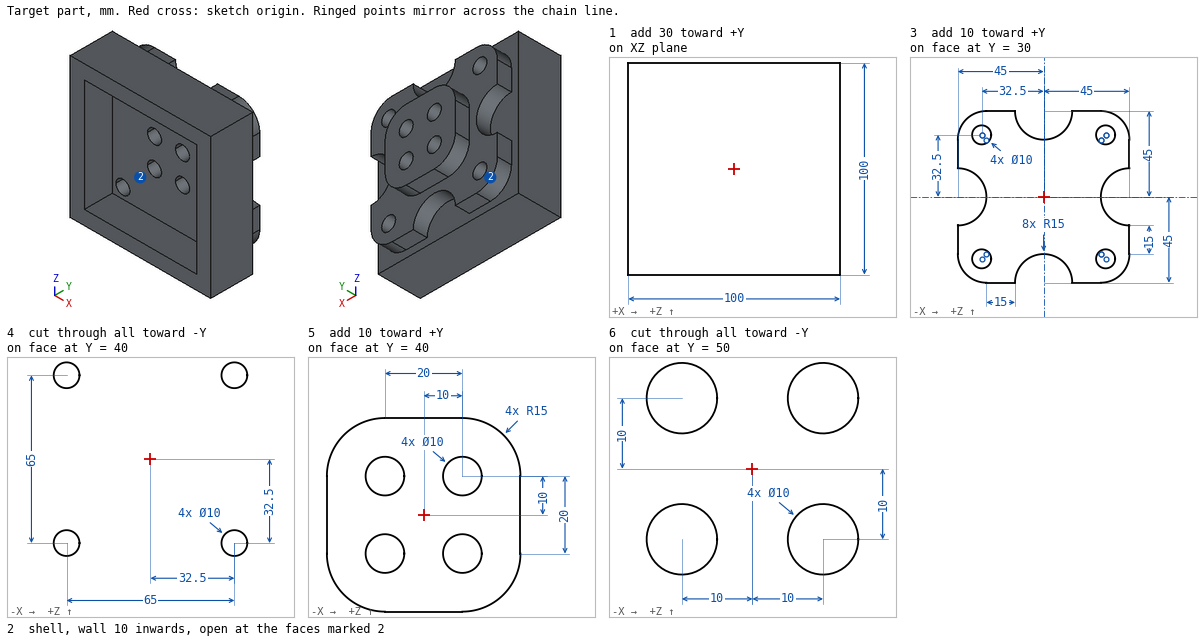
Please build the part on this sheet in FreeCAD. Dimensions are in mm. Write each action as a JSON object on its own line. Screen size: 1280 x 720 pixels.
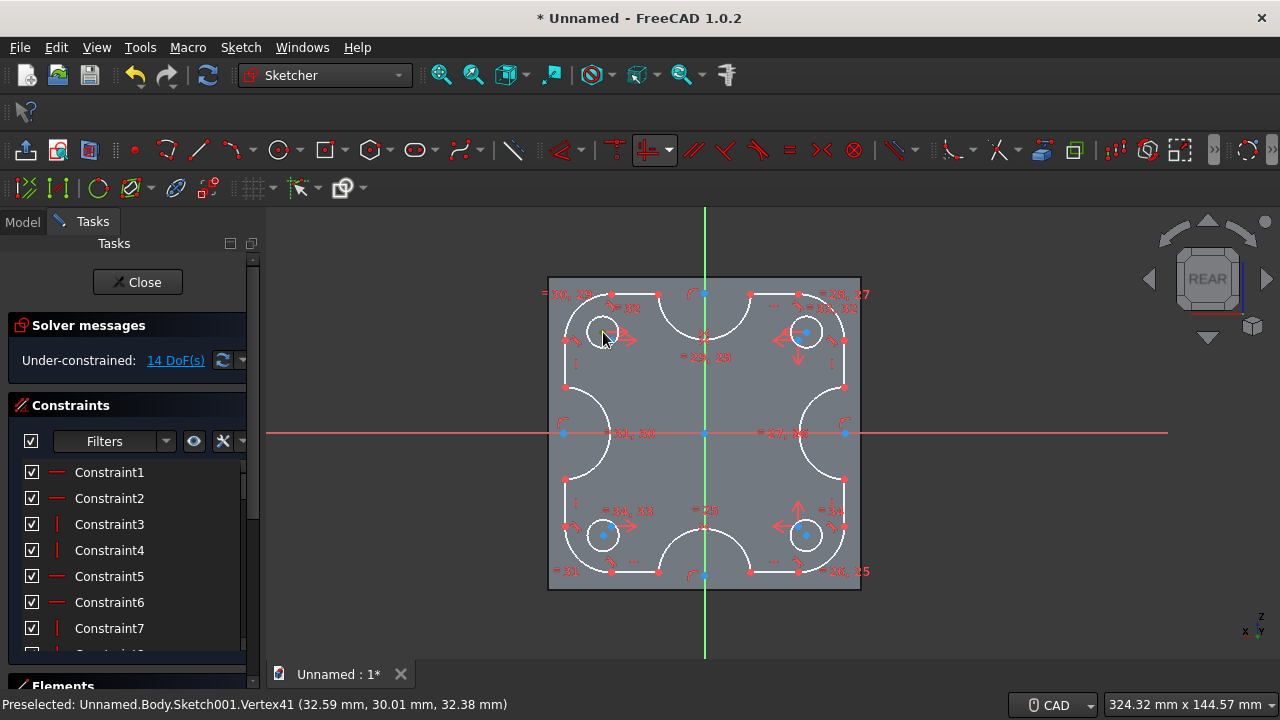
{"action": "left_click", "coordinate": [603, 536]}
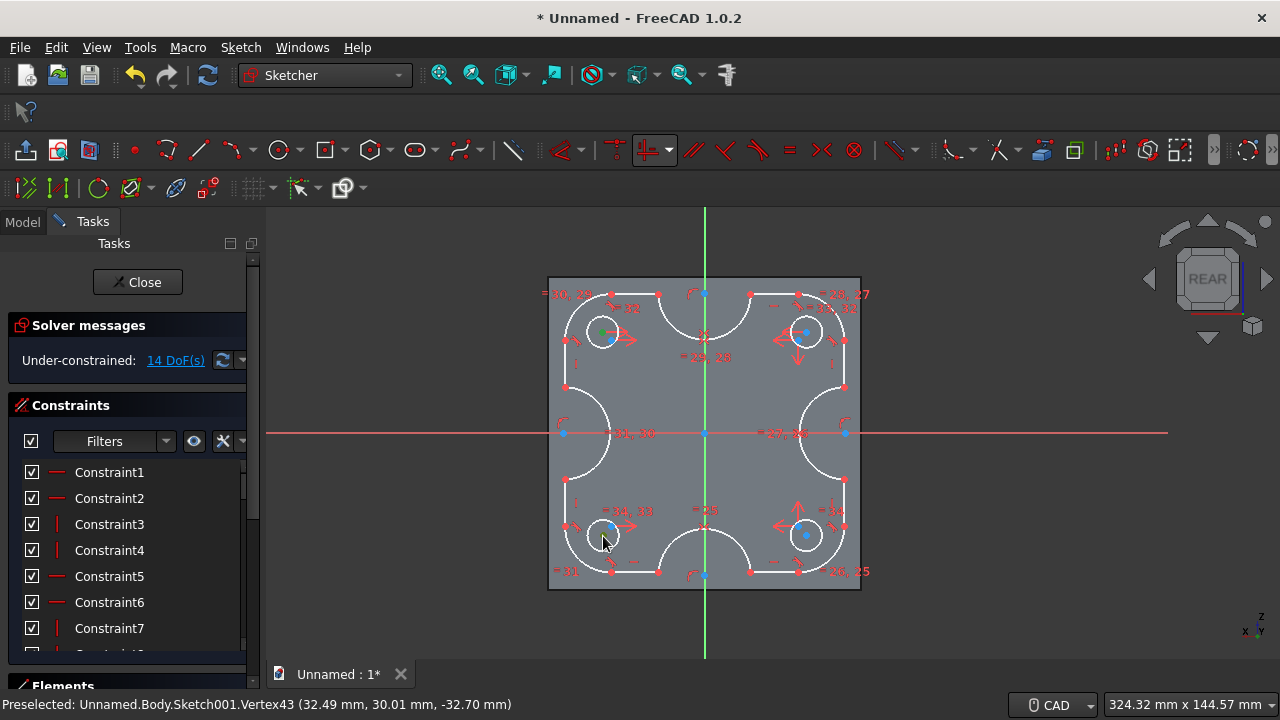
{"action": "left_click", "coordinate": [353, 433]}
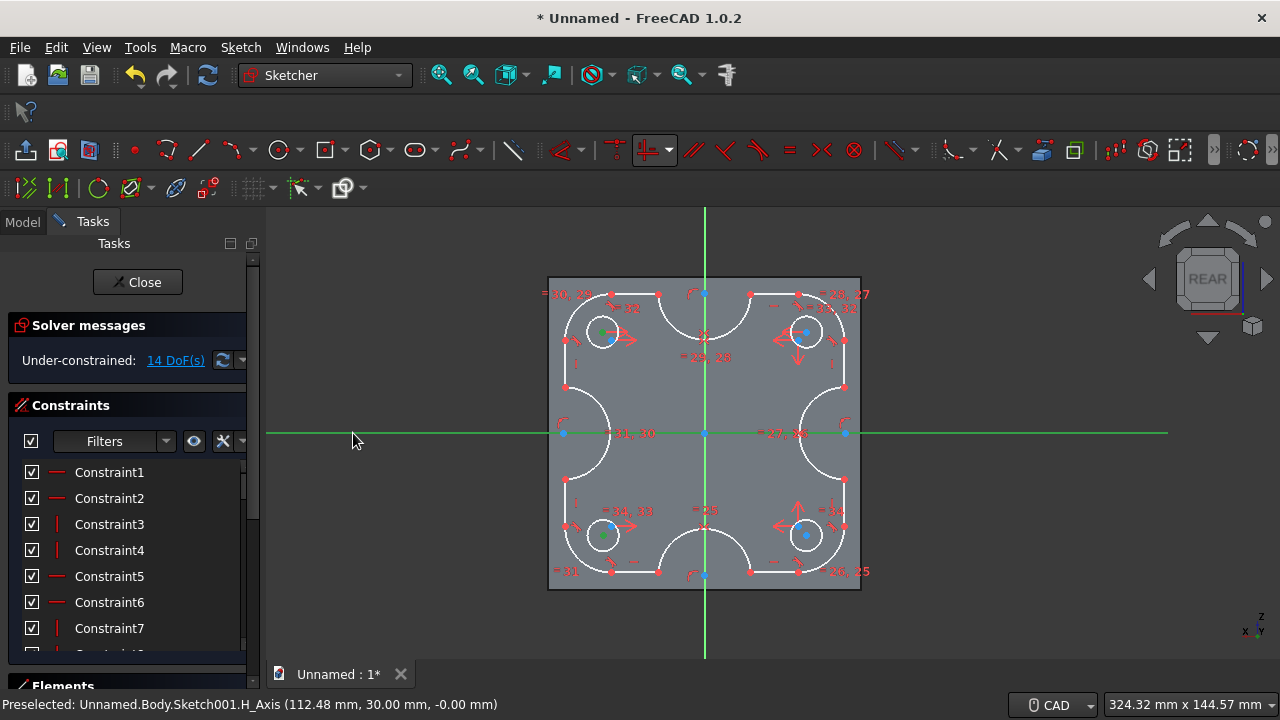
{"action": "left_click", "coordinate": [822, 150]}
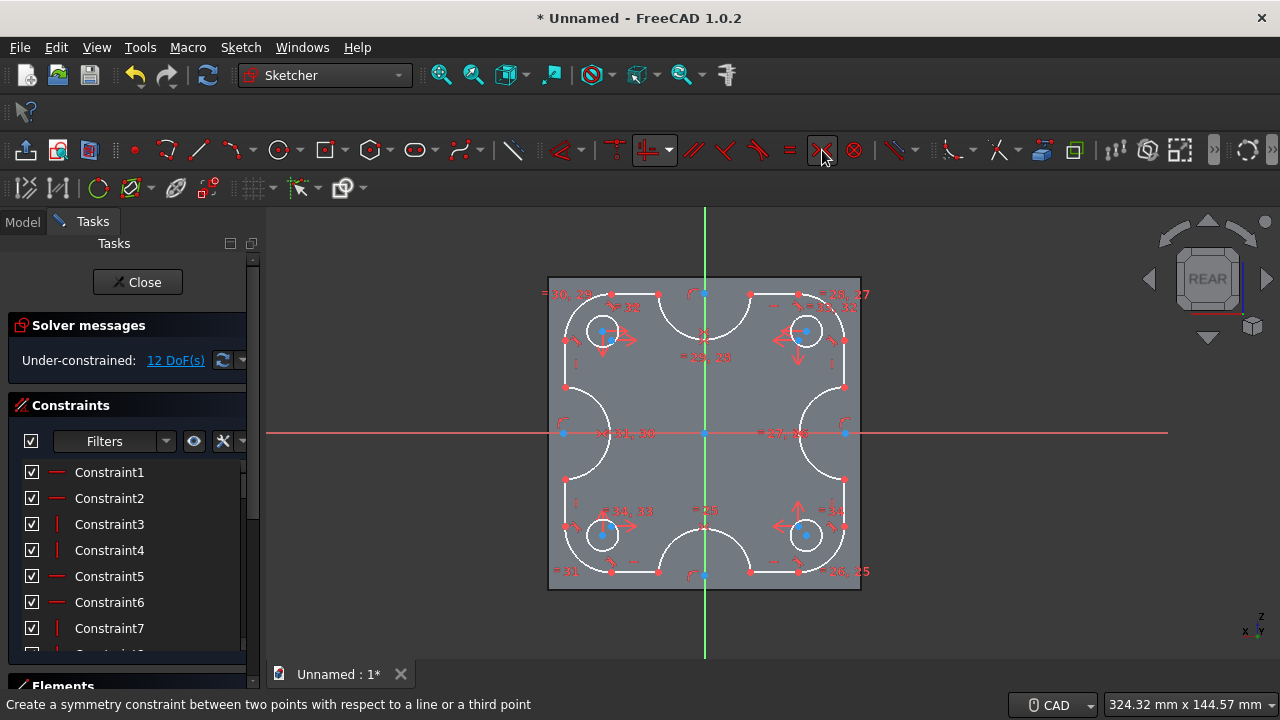
{"action": "left_click", "coordinate": [807, 331]}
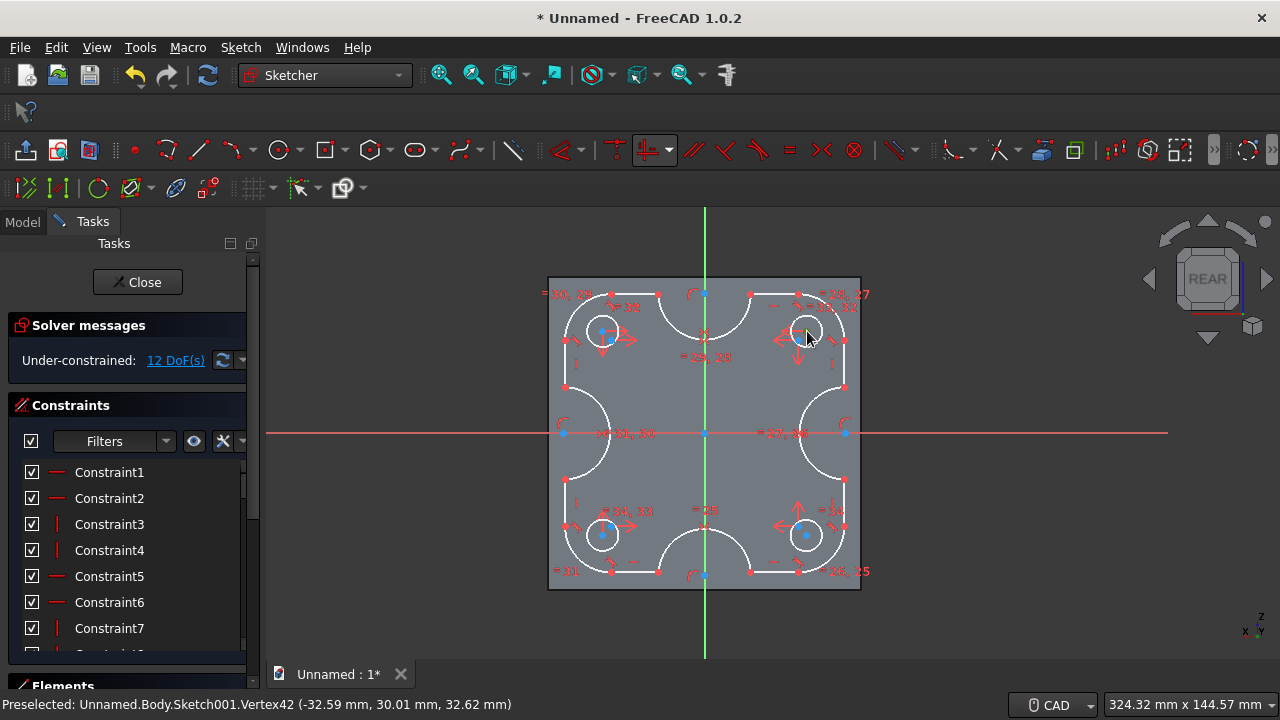
{"action": "left_click", "coordinate": [806, 536]}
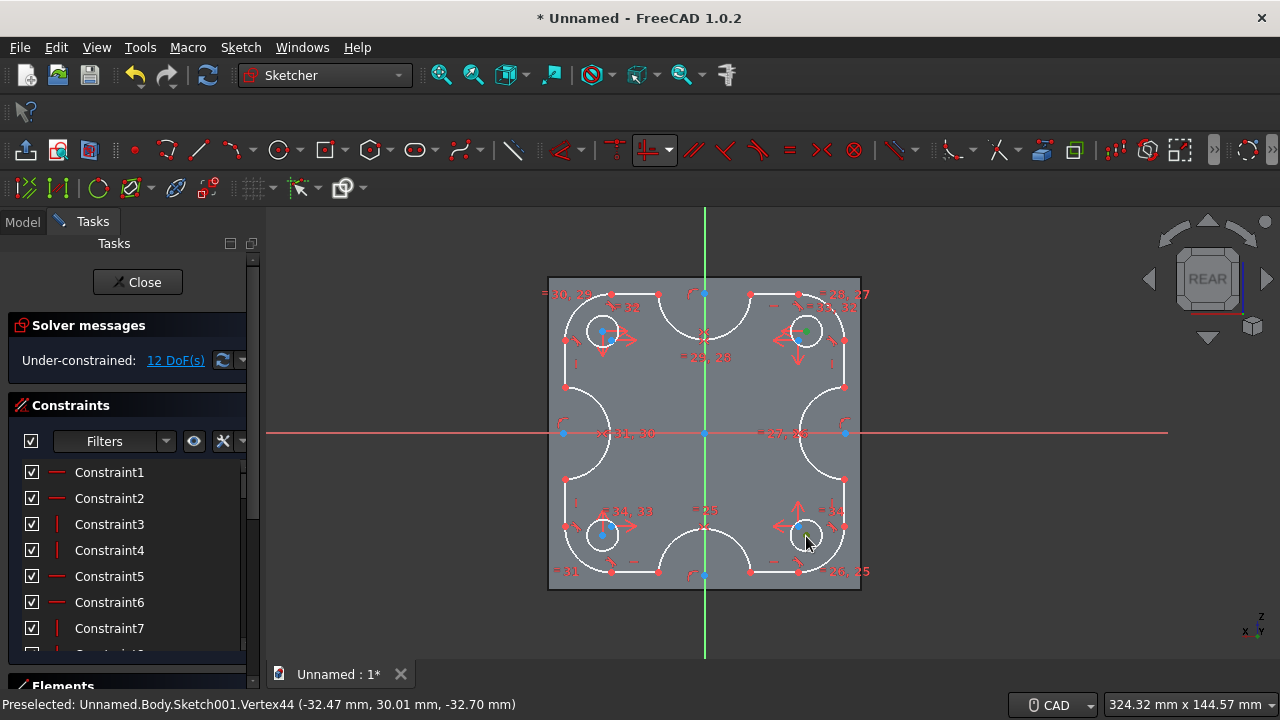
{"action": "left_click", "coordinate": [353, 433]}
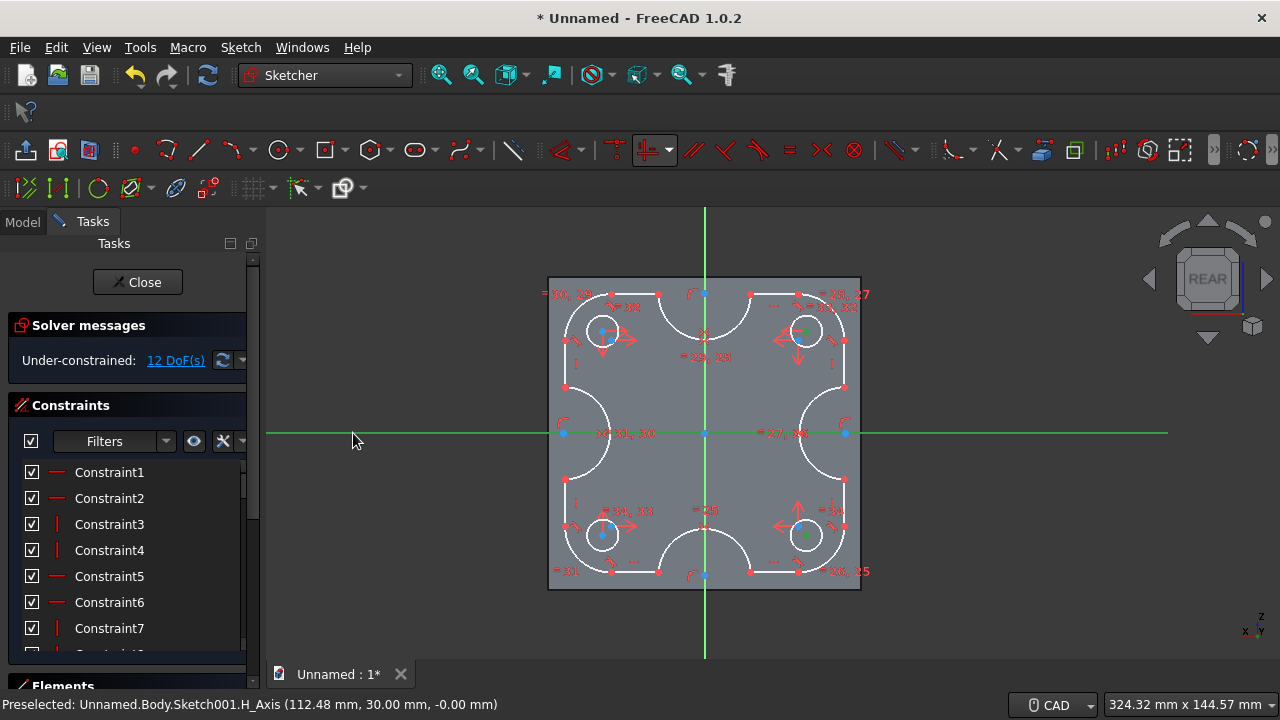
{"action": "left_click", "coordinate": [822, 150]}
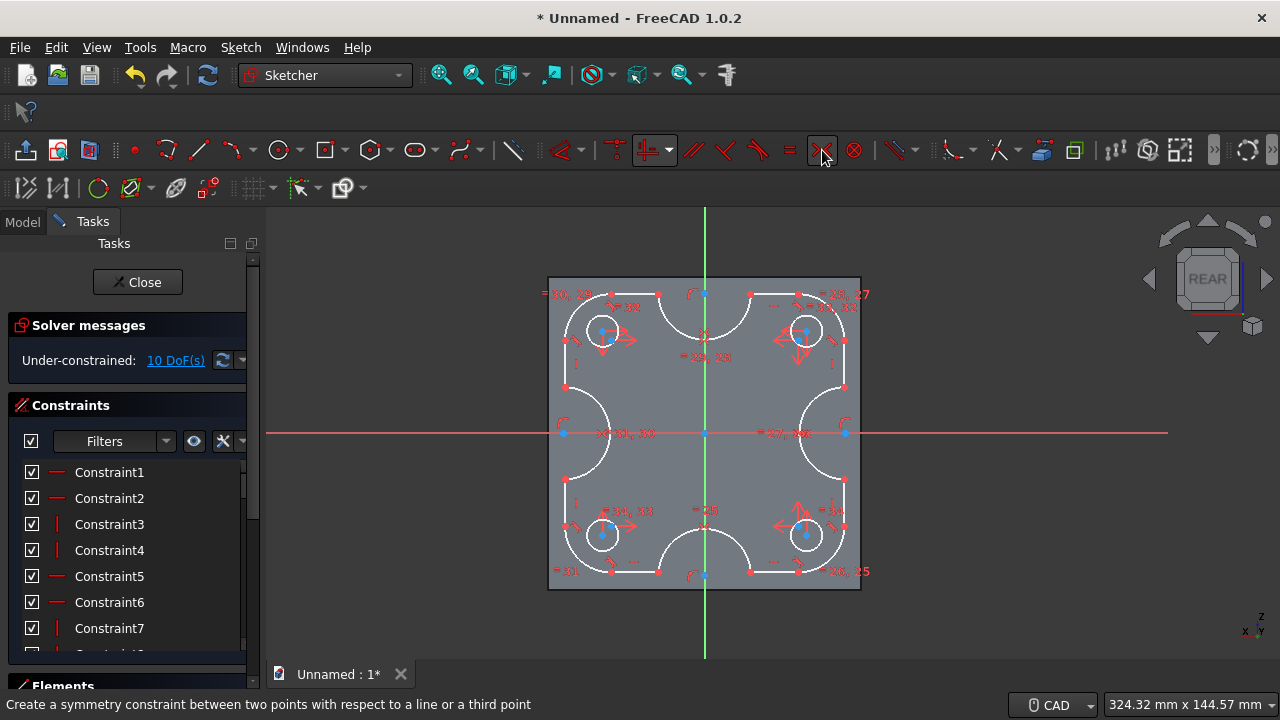
{"action": "left_click", "coordinate": [560, 150]}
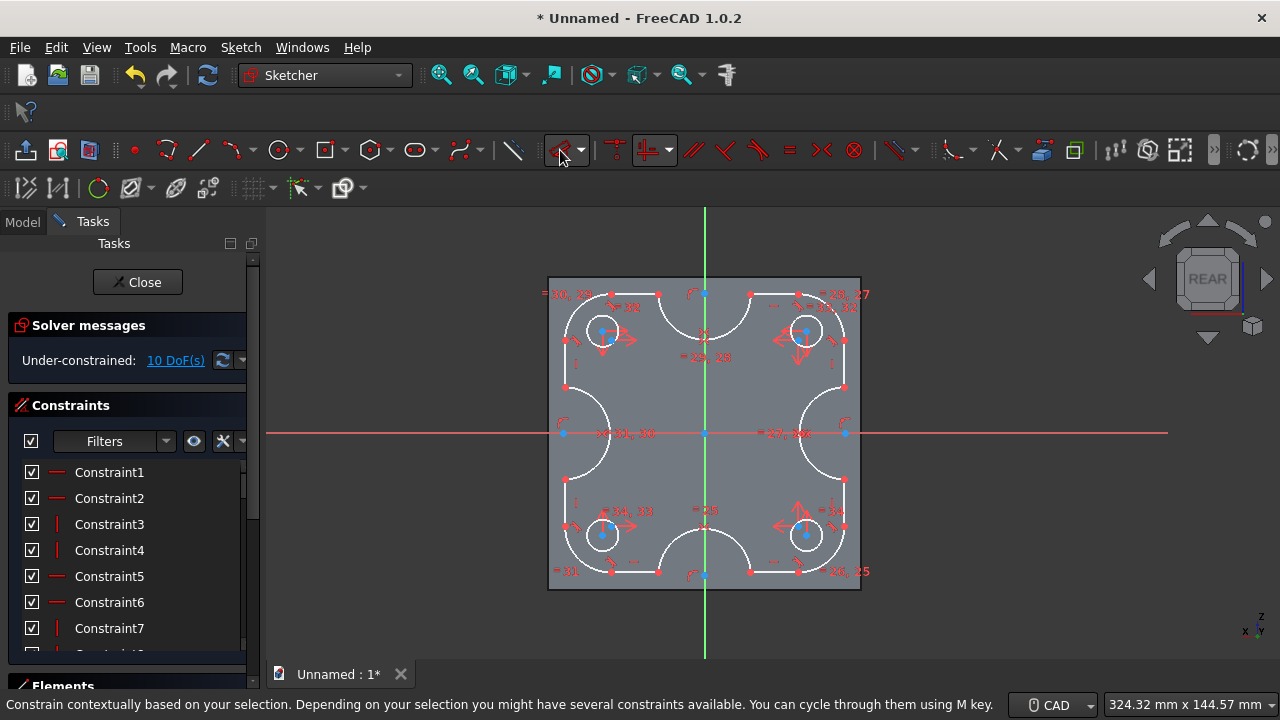
{"action": "left_click", "coordinate": [731, 537]}
{"action": "left_click", "coordinate": [749, 511]}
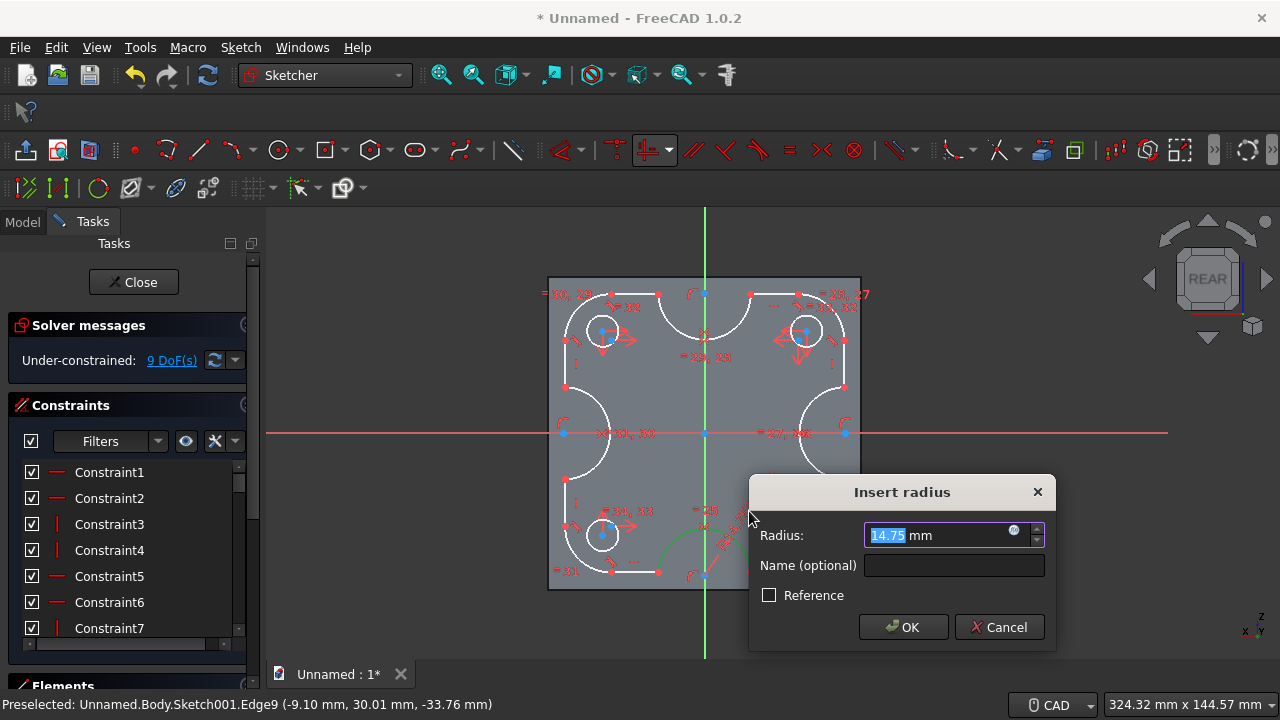
{"action": "type", "text": "15"}
{"action": "key", "text": "Return"}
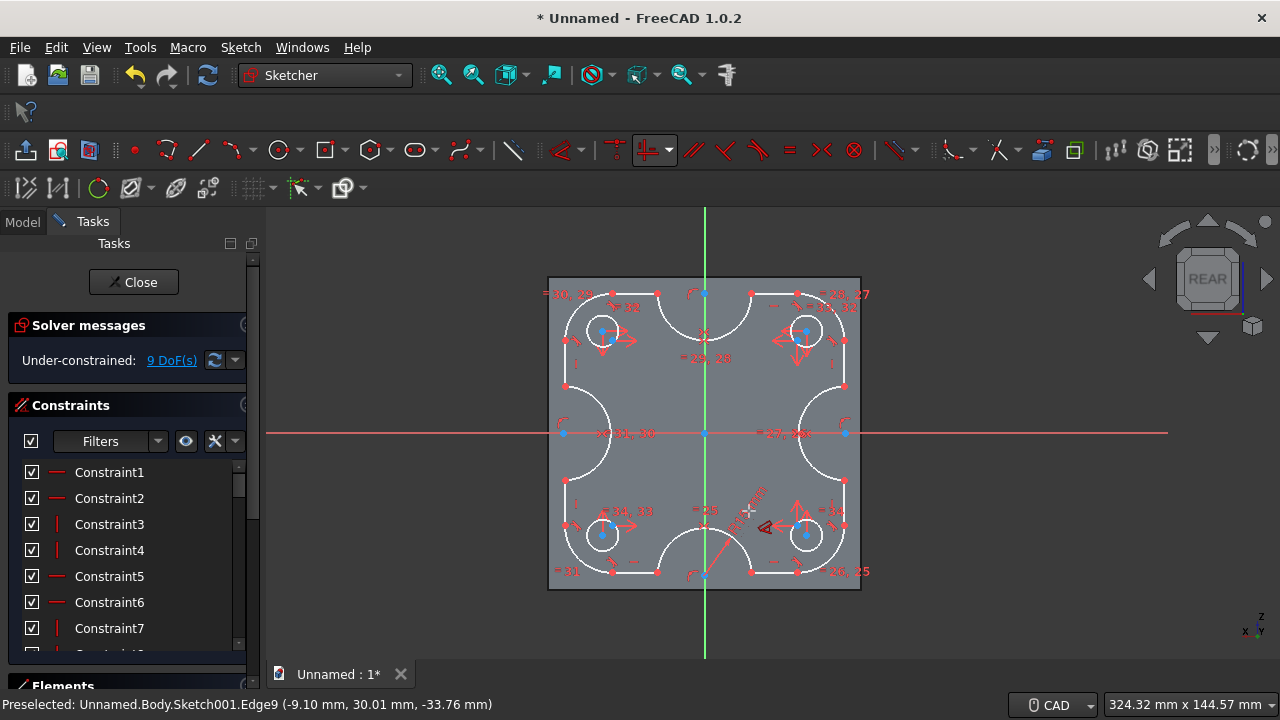
{"action": "scroll", "coordinate": [614, 320], "scroll_direction": "up", "scroll_amount": 2}